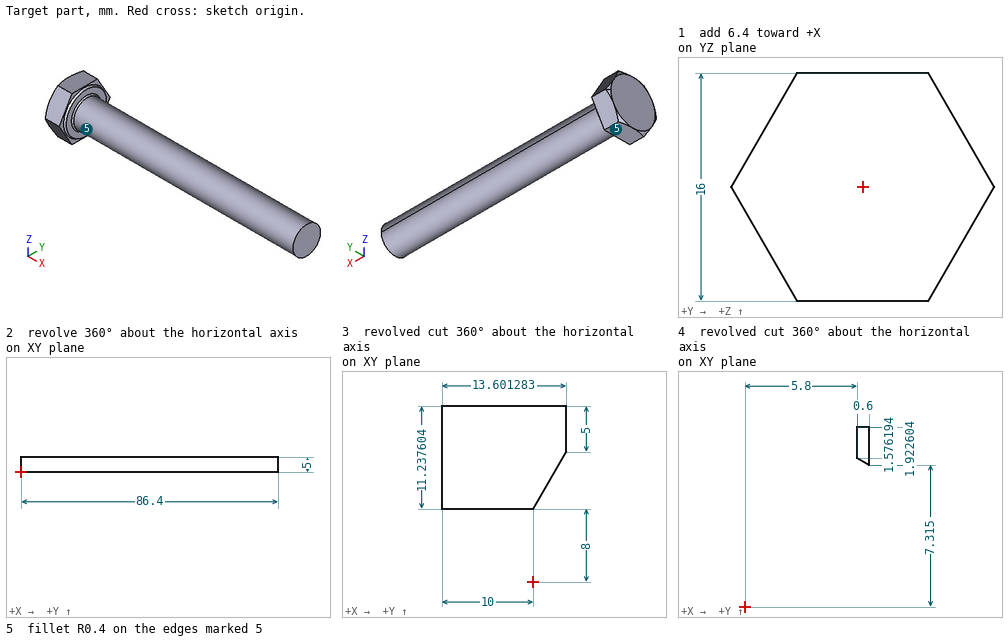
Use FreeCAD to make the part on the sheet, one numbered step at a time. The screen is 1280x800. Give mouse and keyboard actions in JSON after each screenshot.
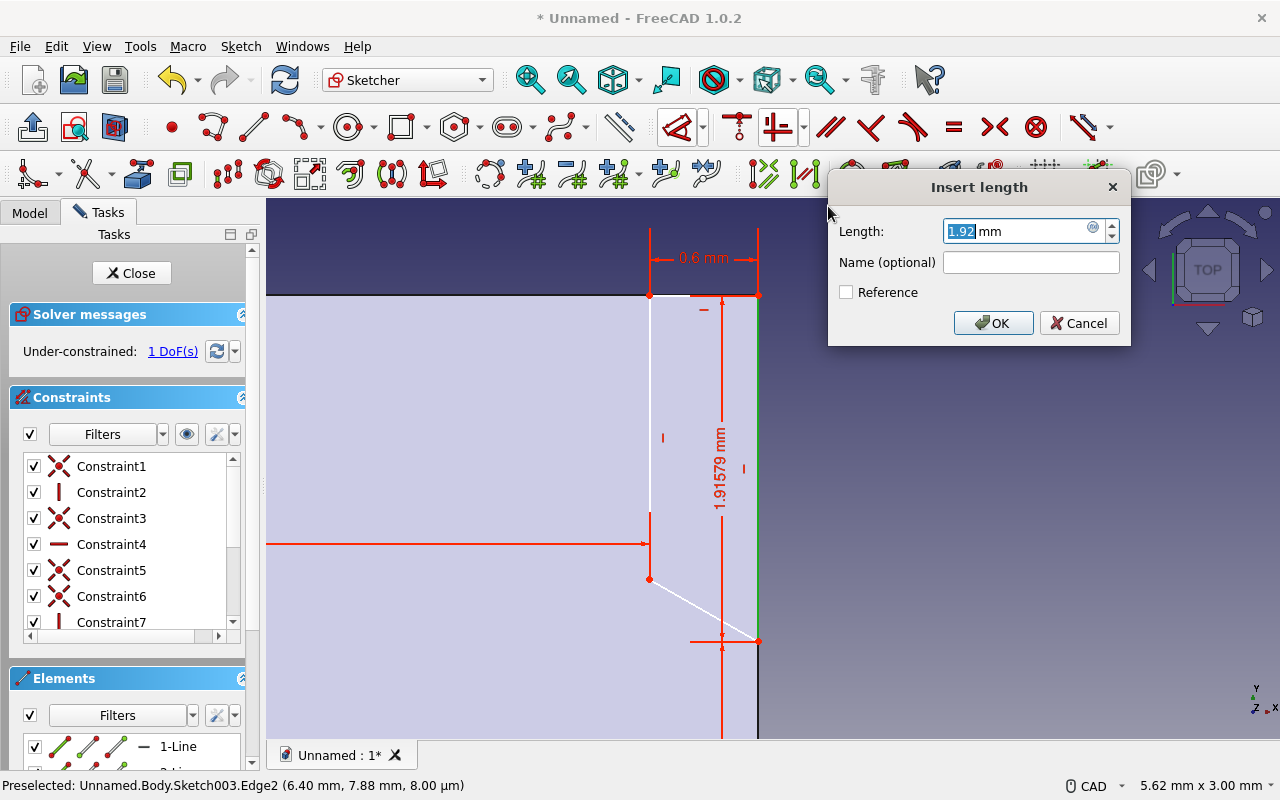
{"action": "type", "text": "1.922604"}
{"action": "key", "text": "Return"}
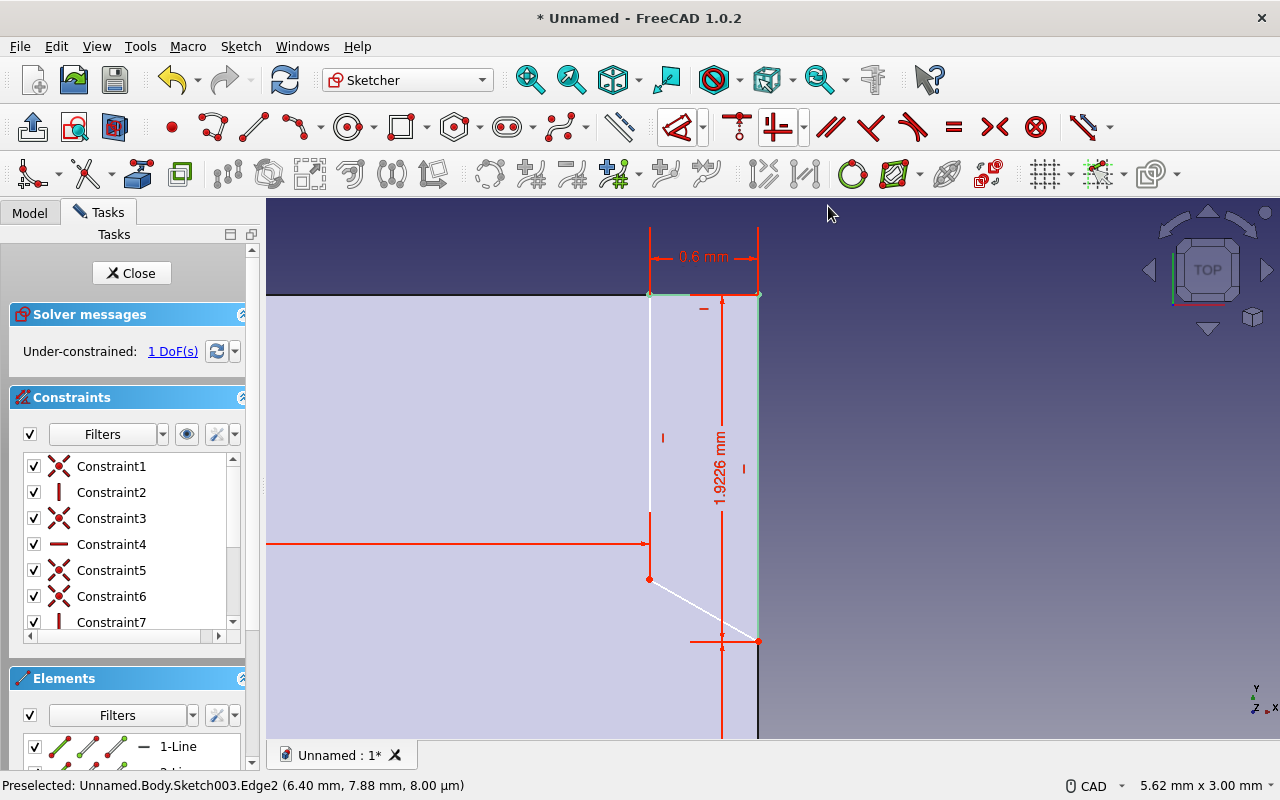
{"action": "left_click", "coordinate": [650, 380]}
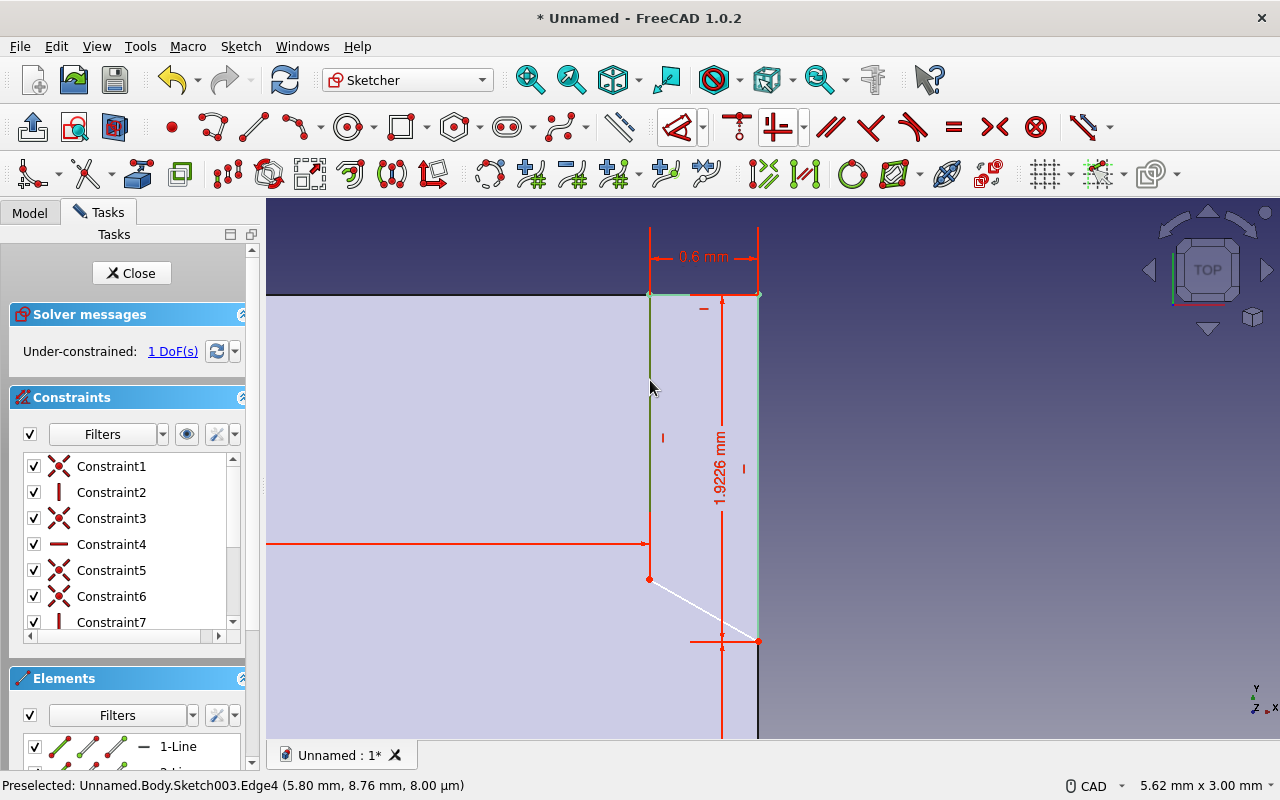
{"action": "key", "text": "i"}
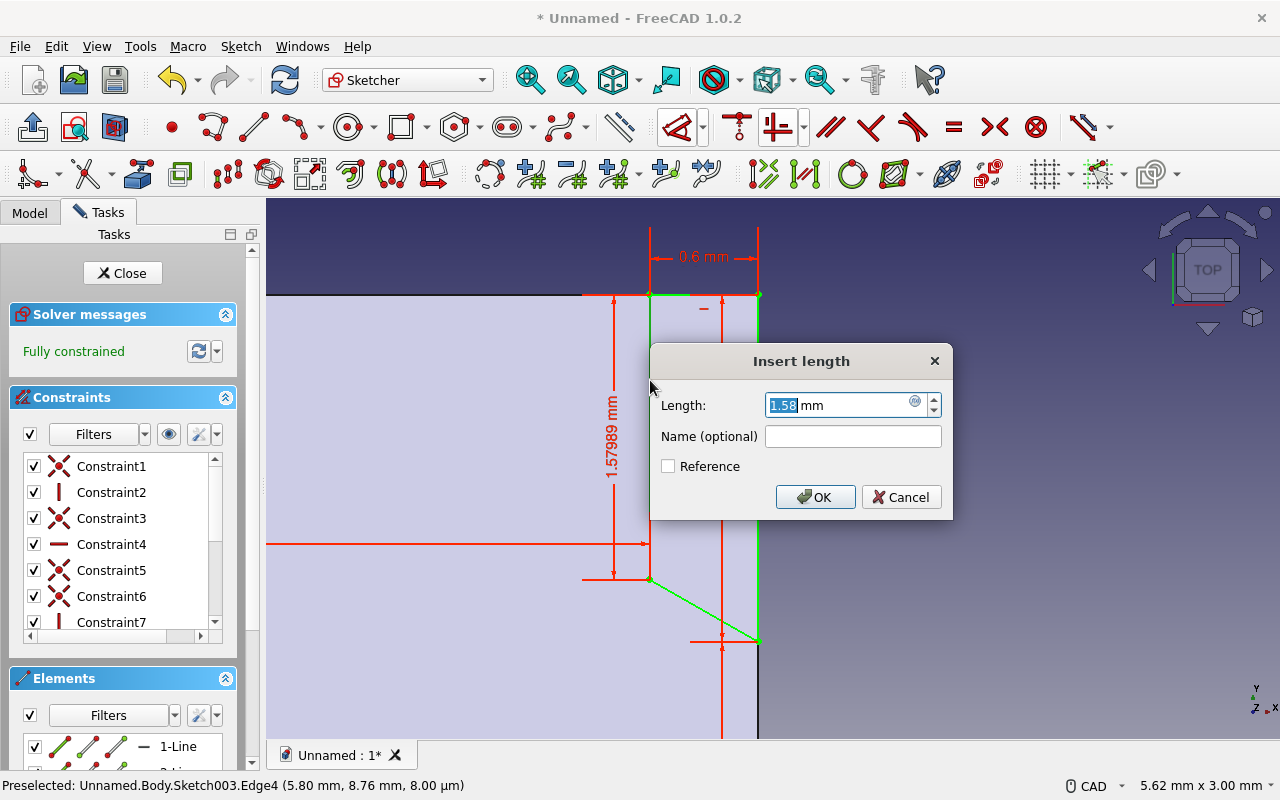
{"action": "type", "text": "1.576194"}
{"action": "key", "text": "Return"}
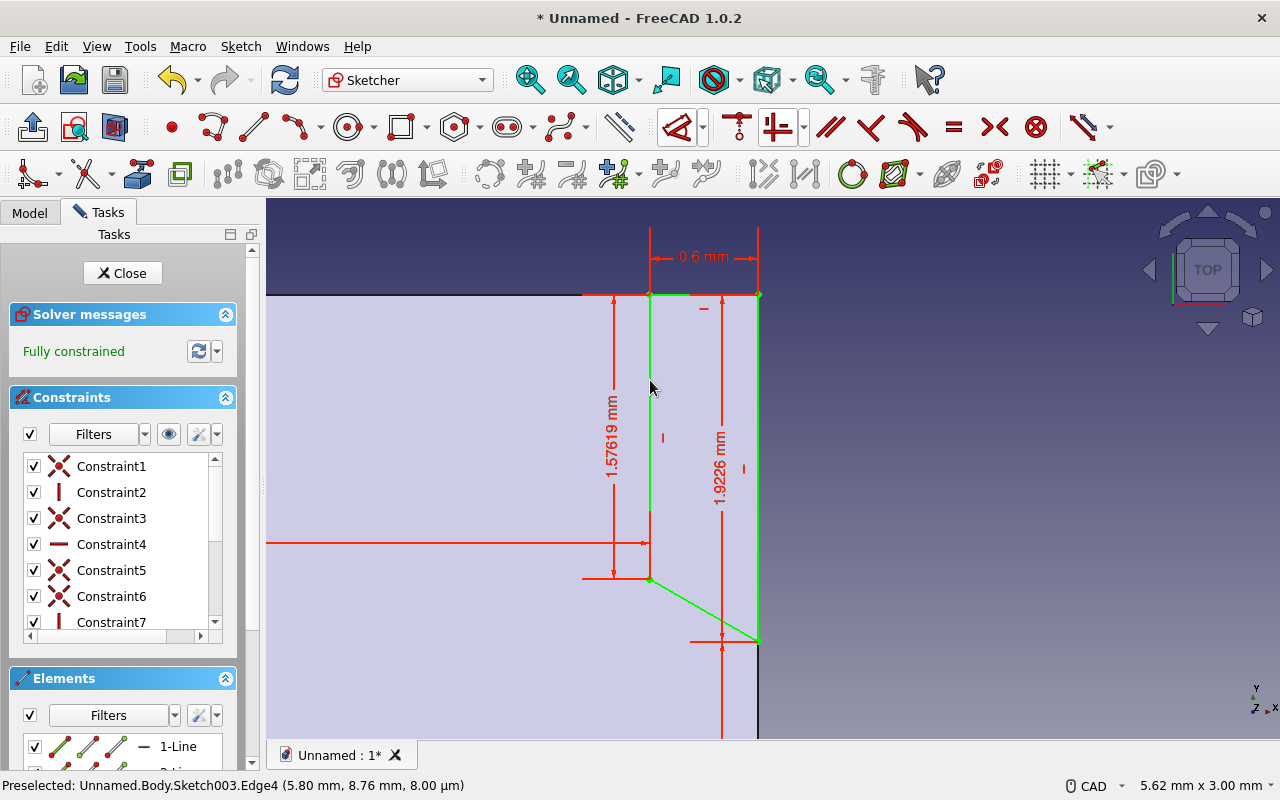
{"action": "left_click", "coordinate": [123, 273]}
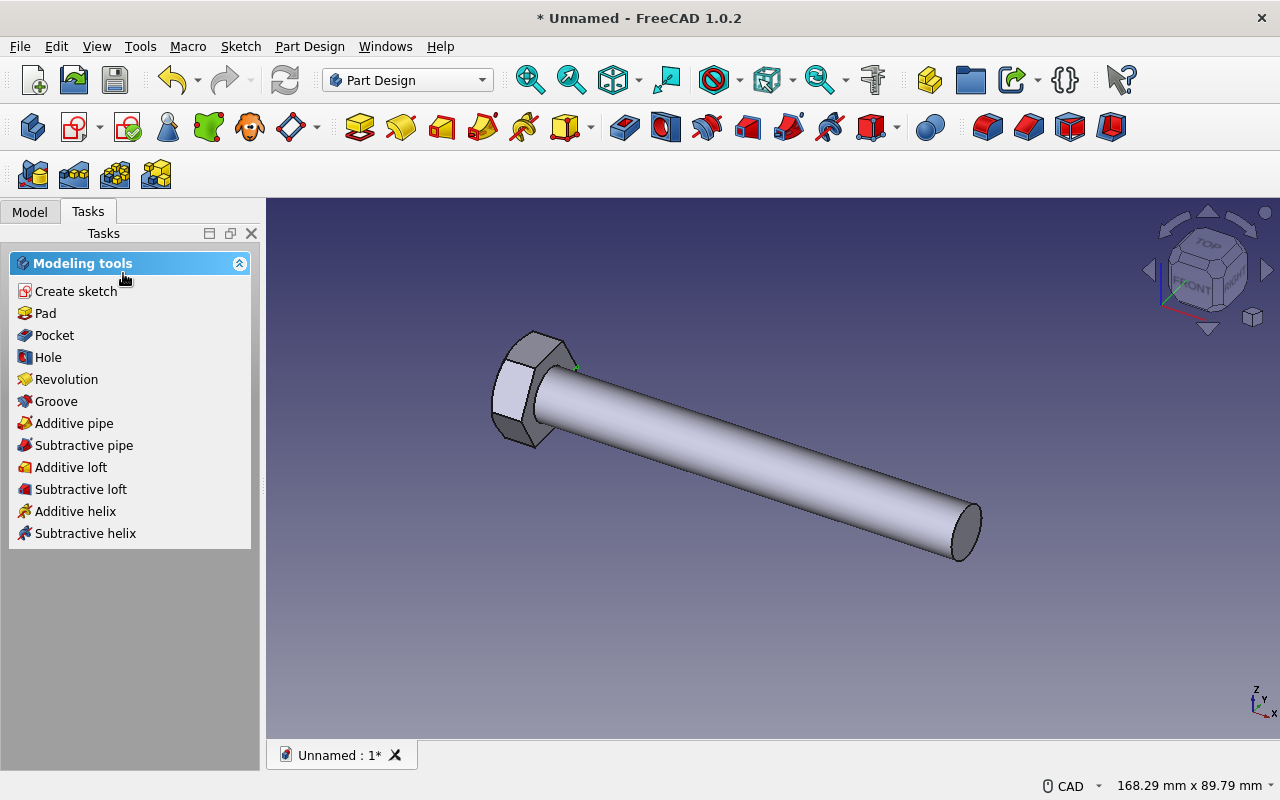
{"action": "left_click", "coordinate": [707, 128]}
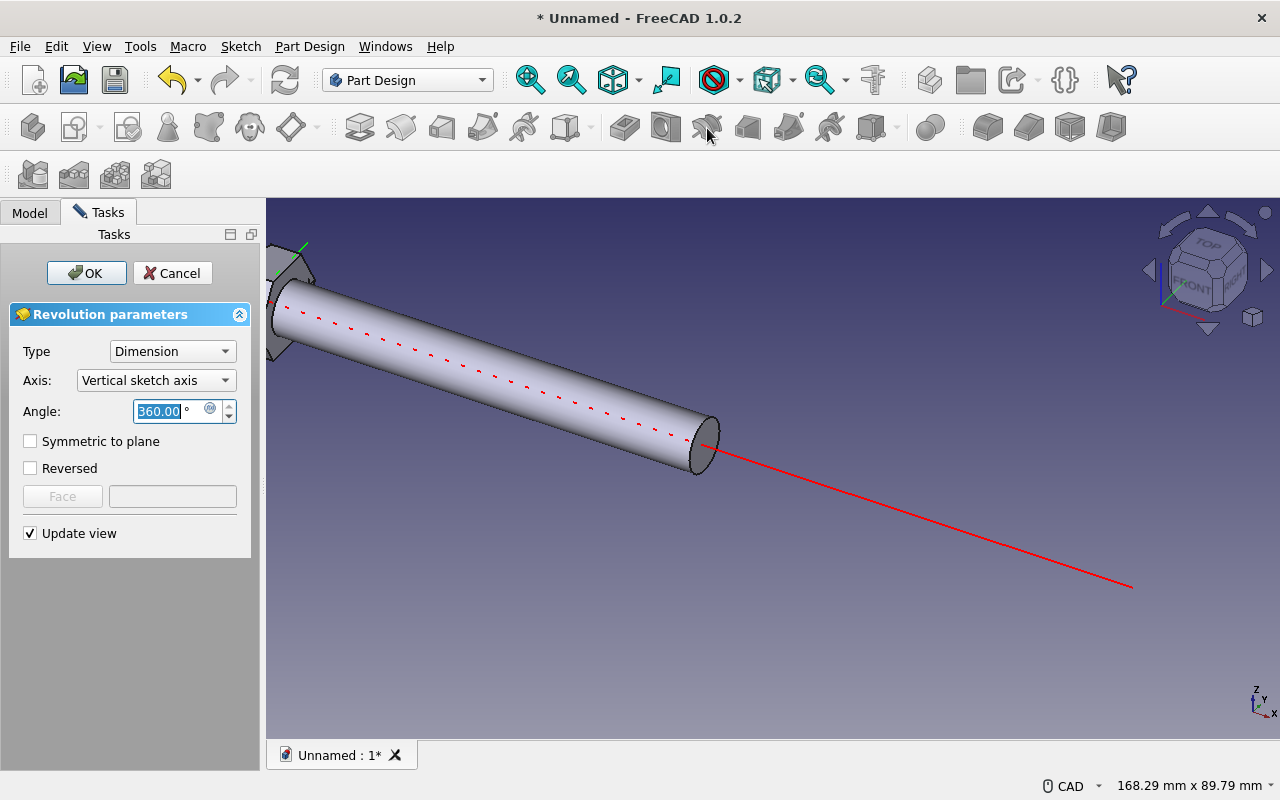
{"action": "left_click", "coordinate": [157, 380]}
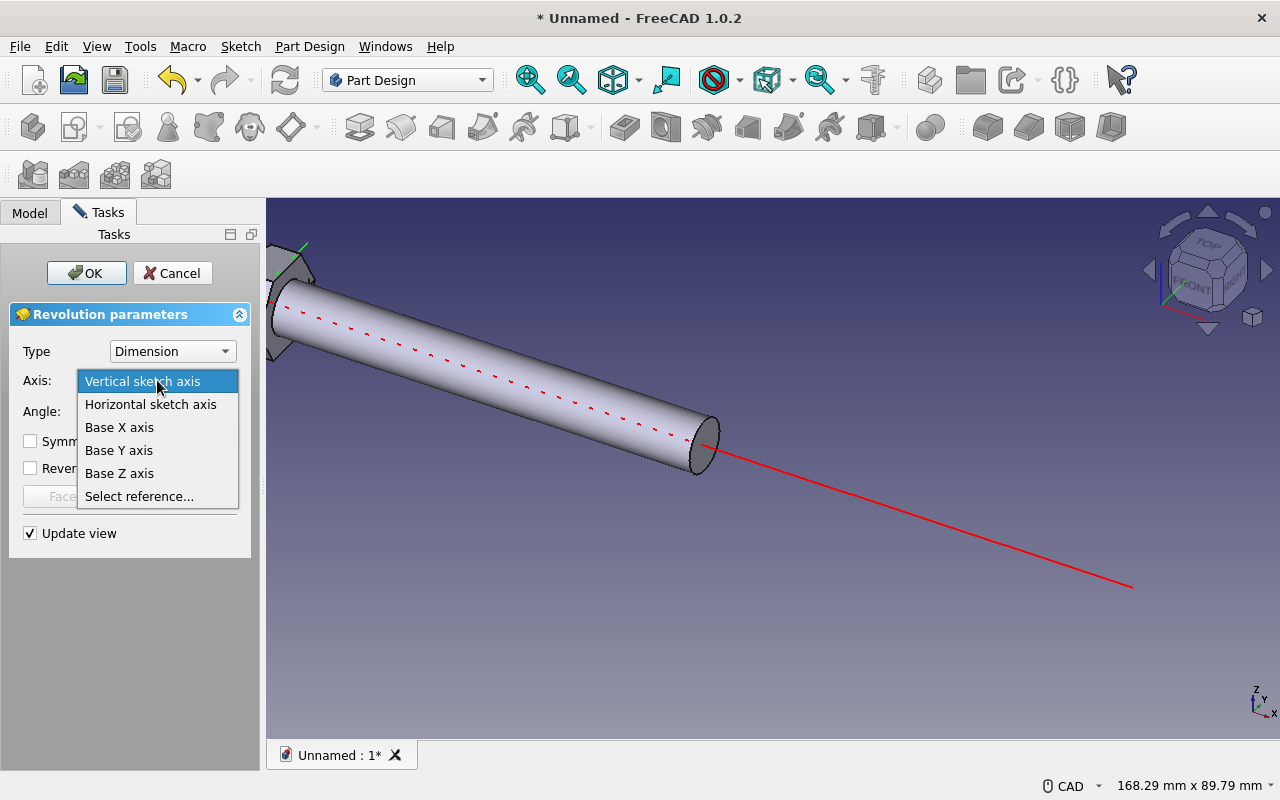
{"action": "left_click", "coordinate": [156, 404]}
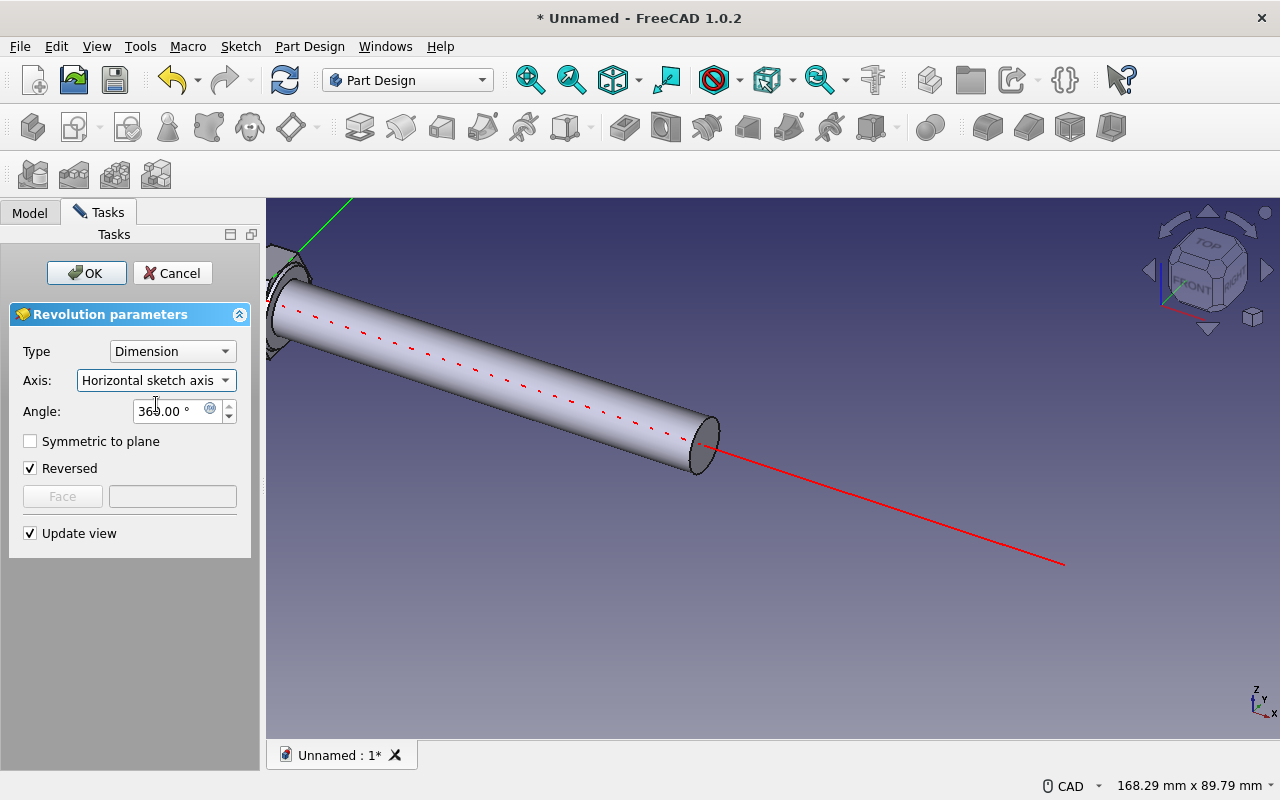
{"action": "left_click", "coordinate": [87, 273]}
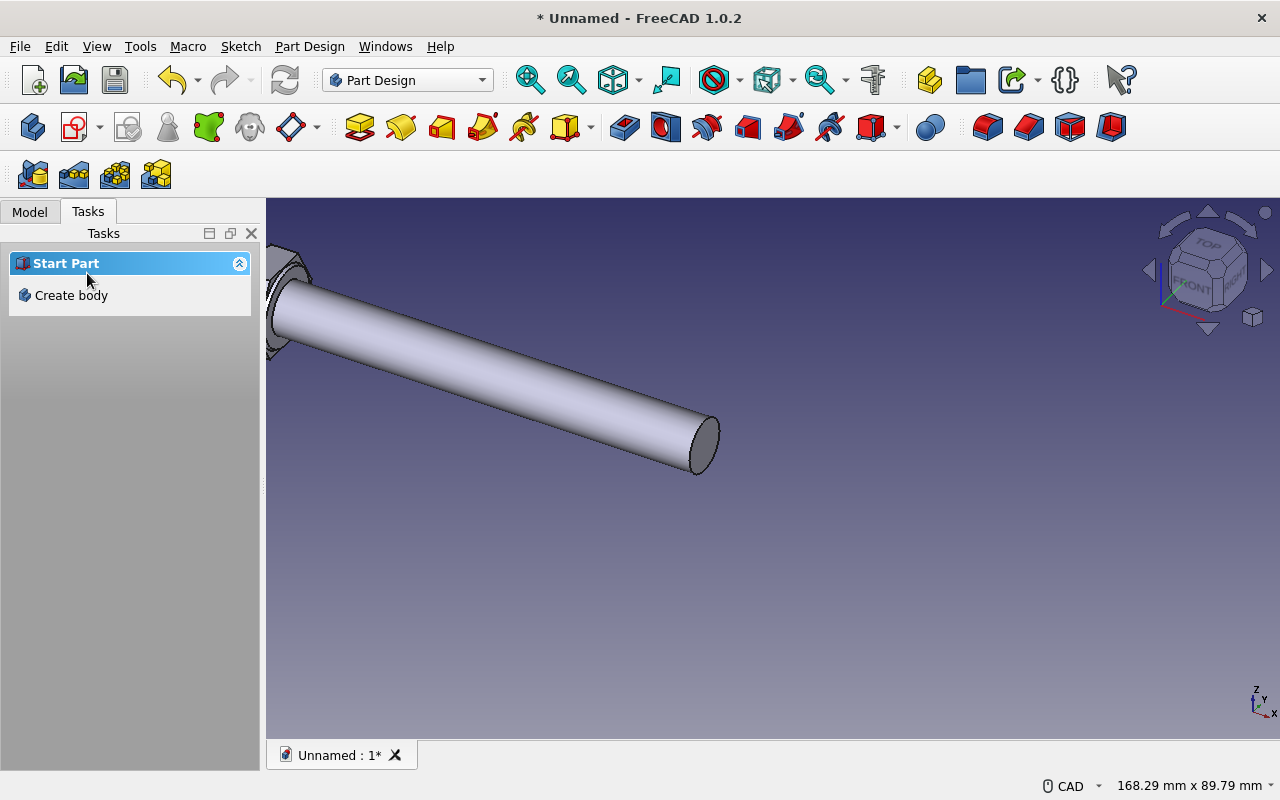
{"action": "left_click", "coordinate": [531, 80]}